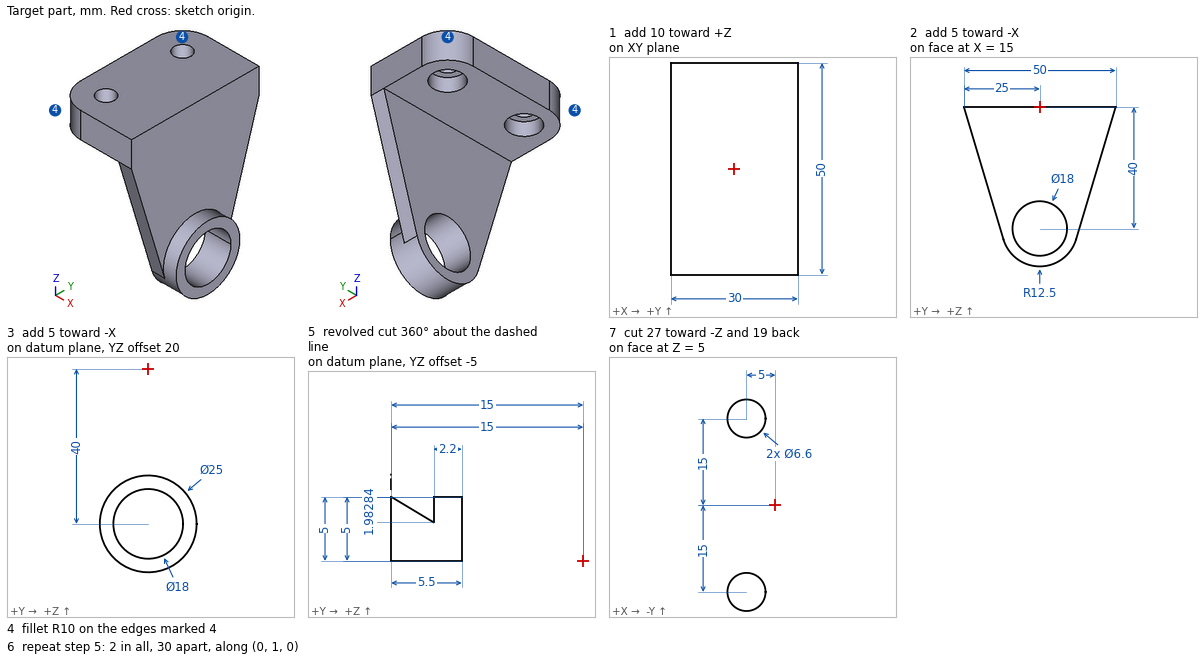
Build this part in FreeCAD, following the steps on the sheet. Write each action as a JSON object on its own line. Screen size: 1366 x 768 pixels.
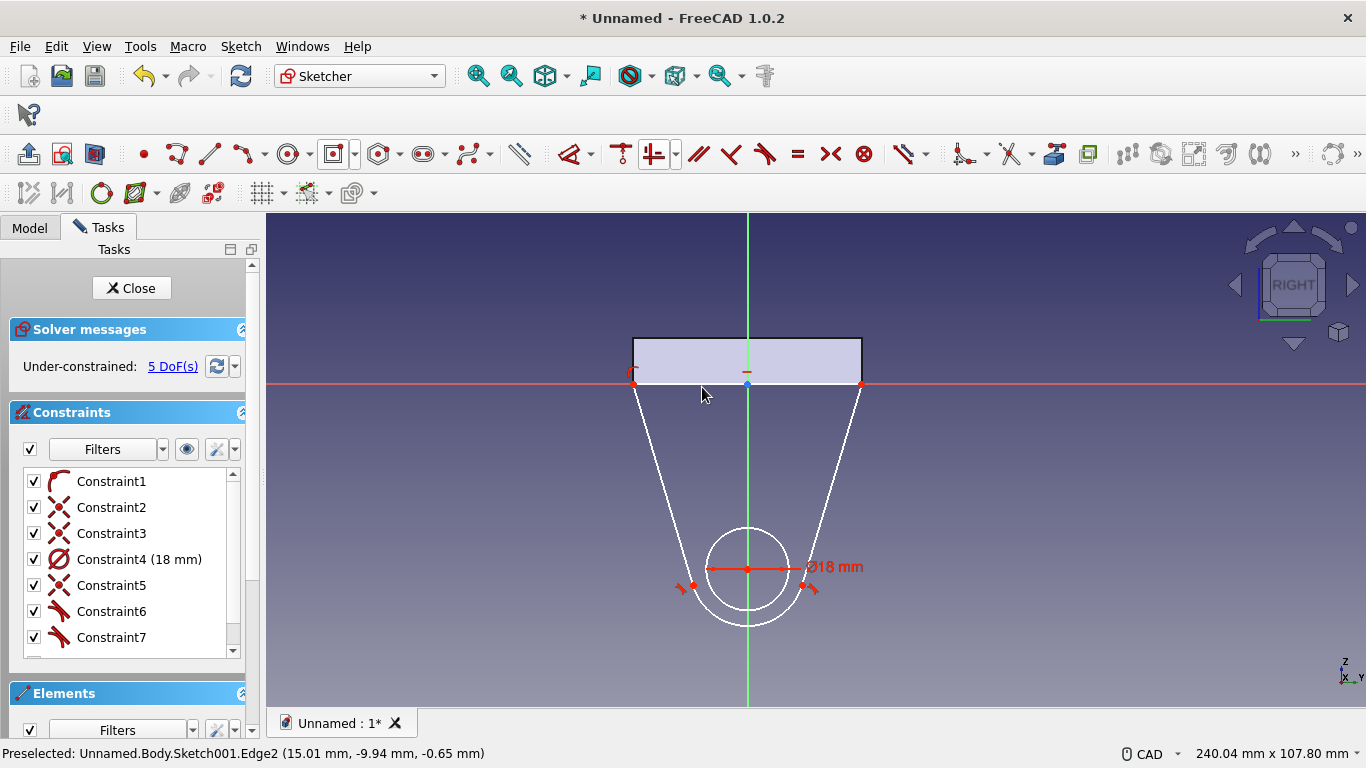
{"action": "left_click", "coordinate": [748, 569]}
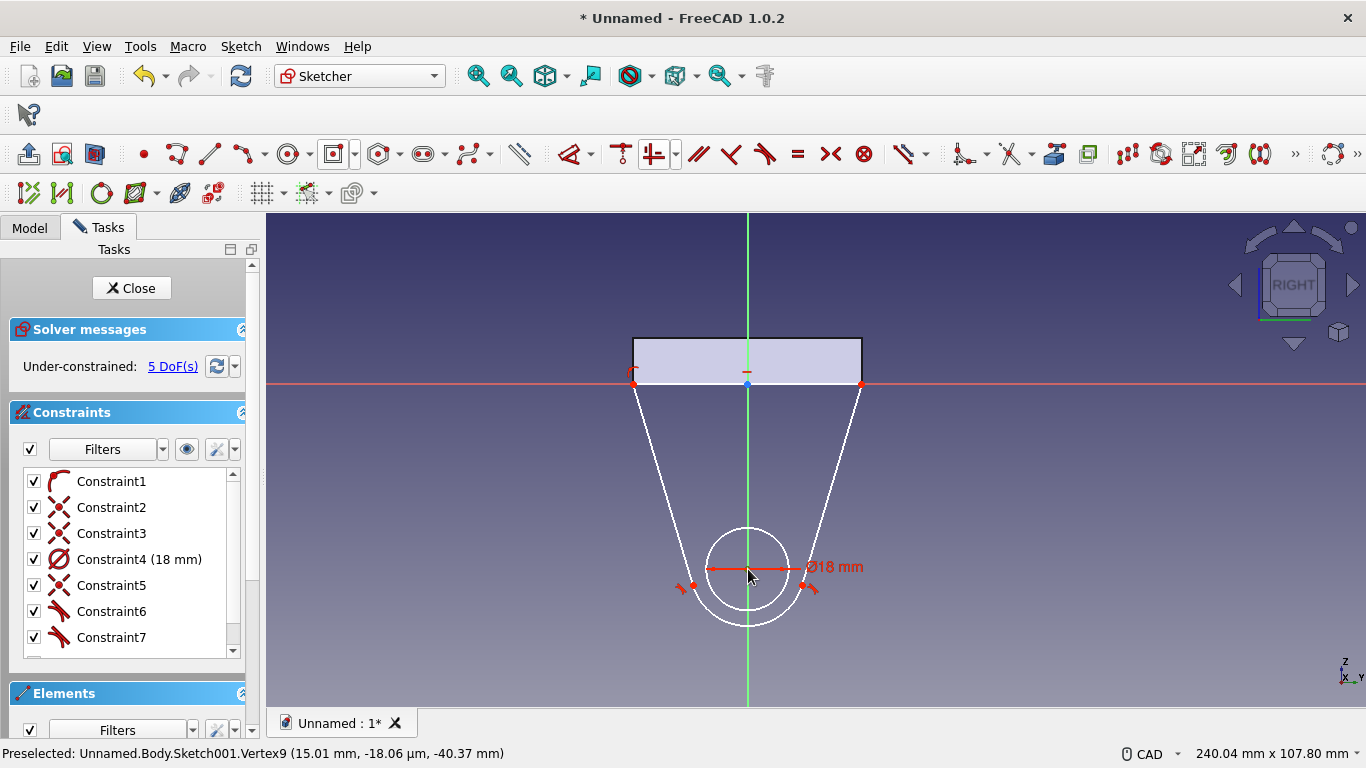
{"action": "left_click", "coordinate": [748, 491]}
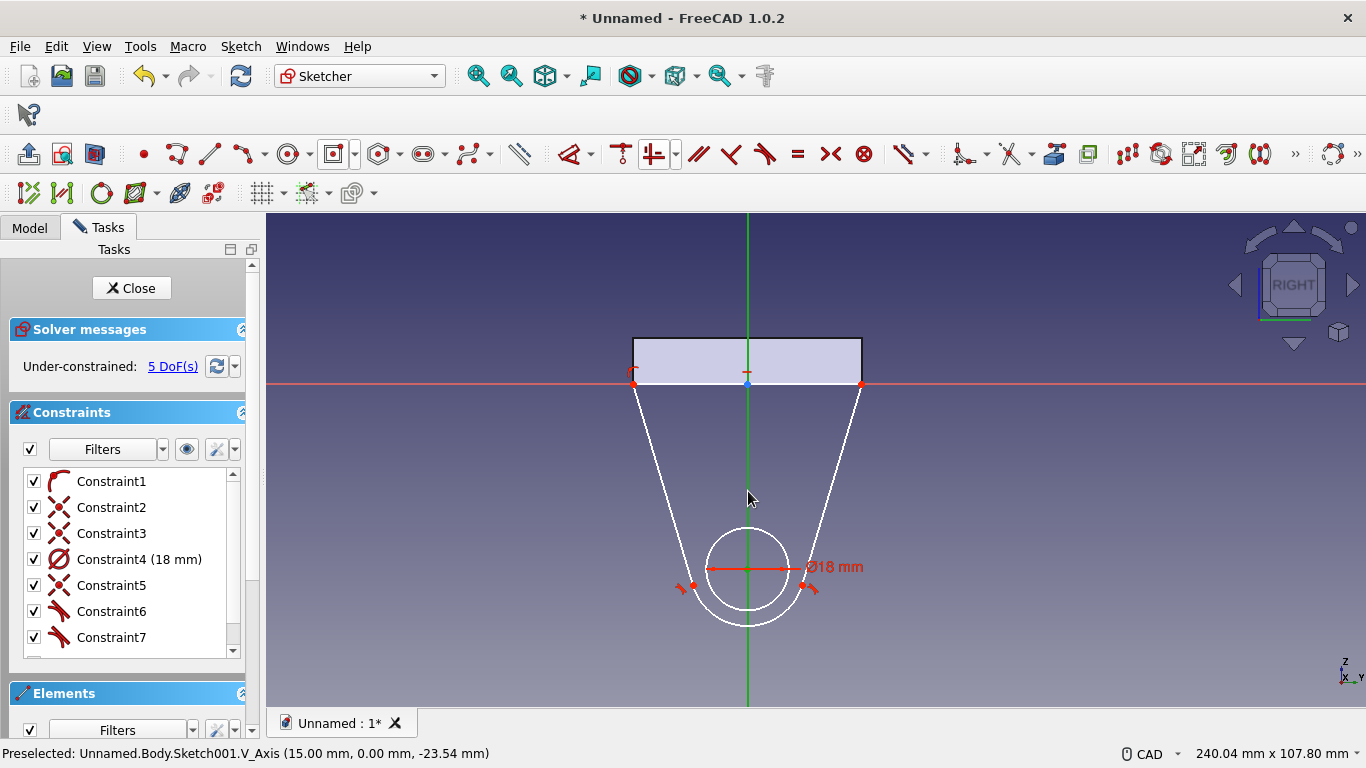
{"action": "left_click", "coordinate": [621, 154]}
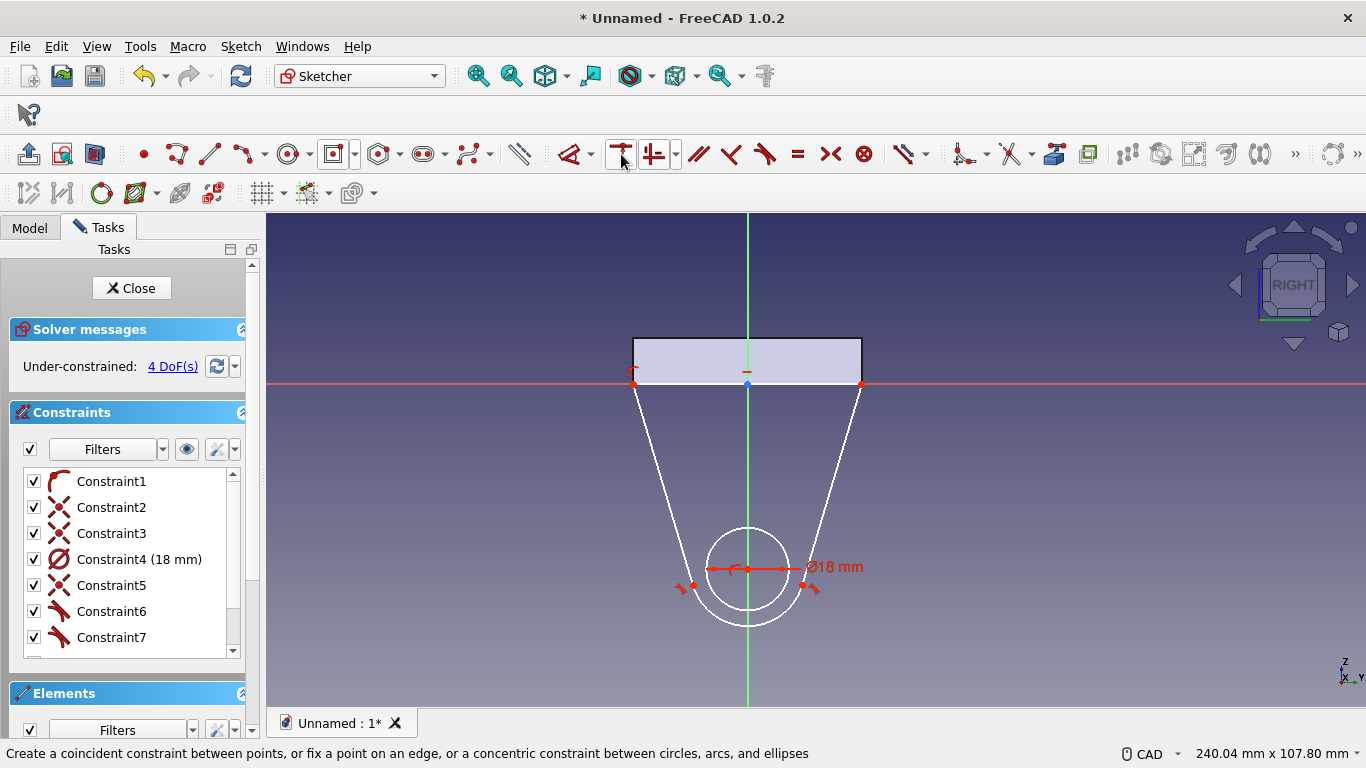
{"action": "left_click", "coordinate": [568, 154]}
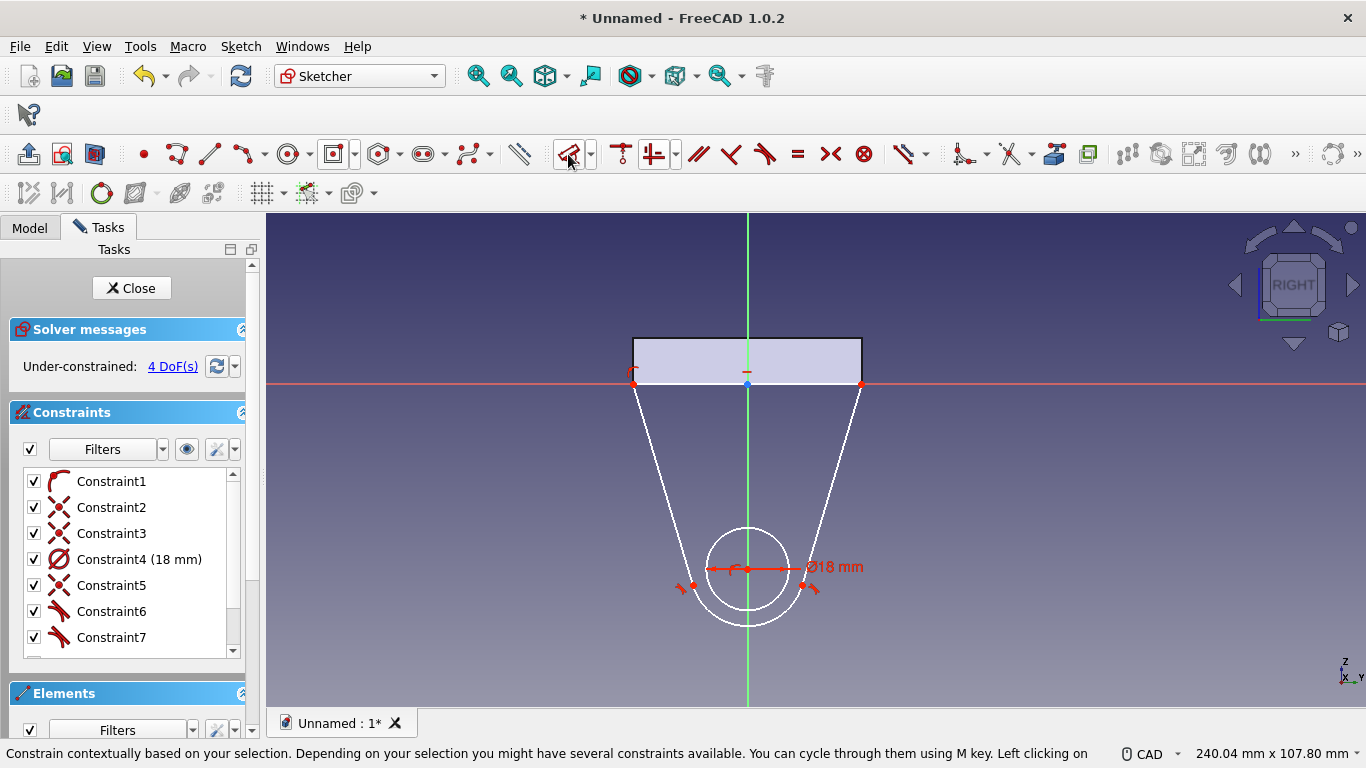
{"action": "left_click", "coordinate": [720, 619]}
{"action": "left_click", "coordinate": [705, 647]}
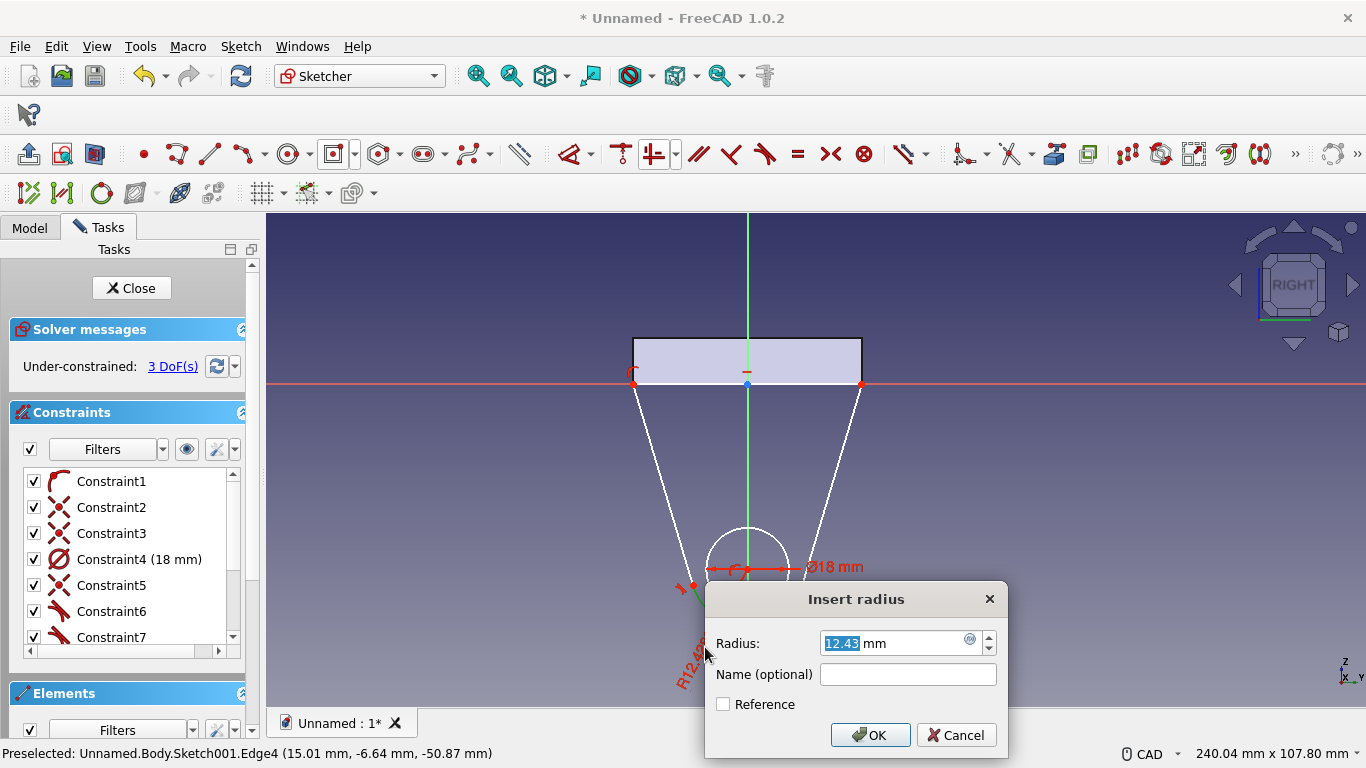
{"action": "type", "text": "12.5"}
{"action": "key", "text": "Return"}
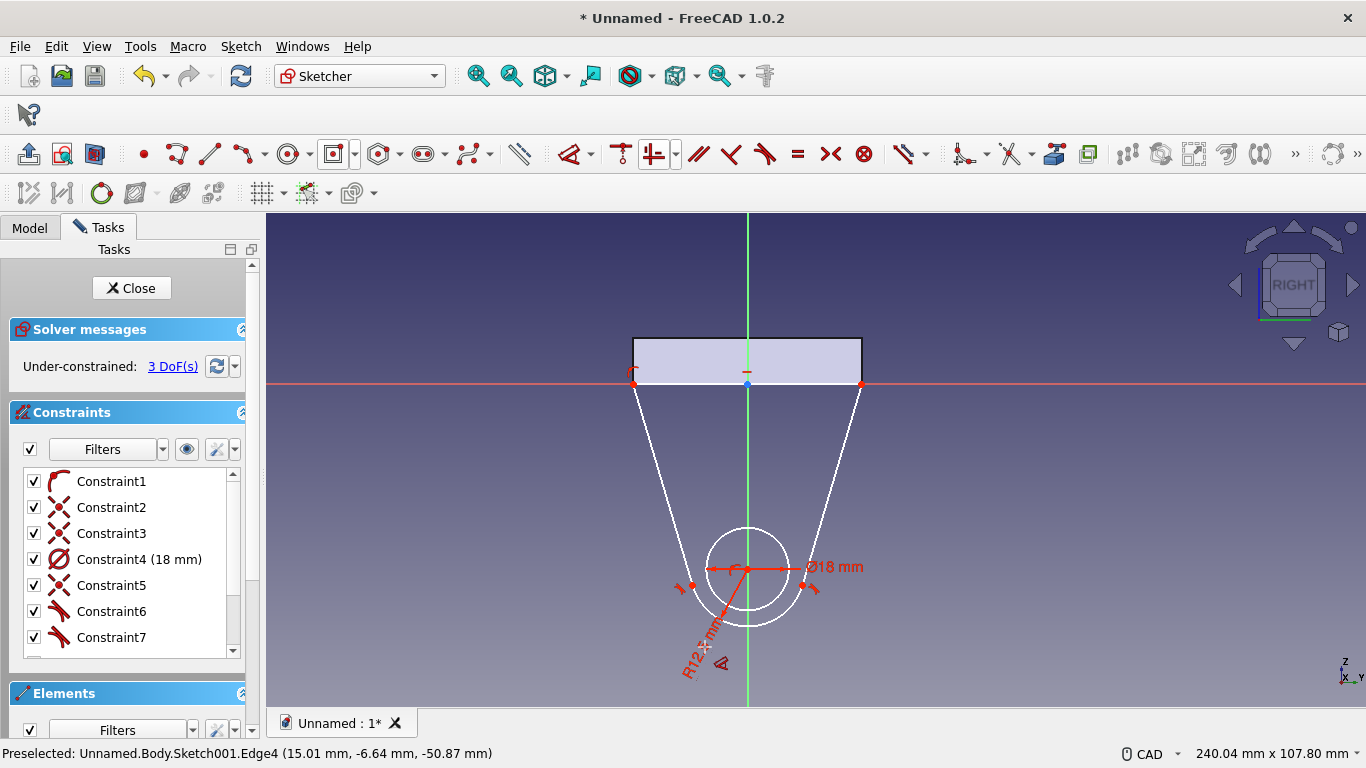
{"action": "left_click", "coordinate": [702, 384]}
{"action": "left_click", "coordinate": [695, 350]}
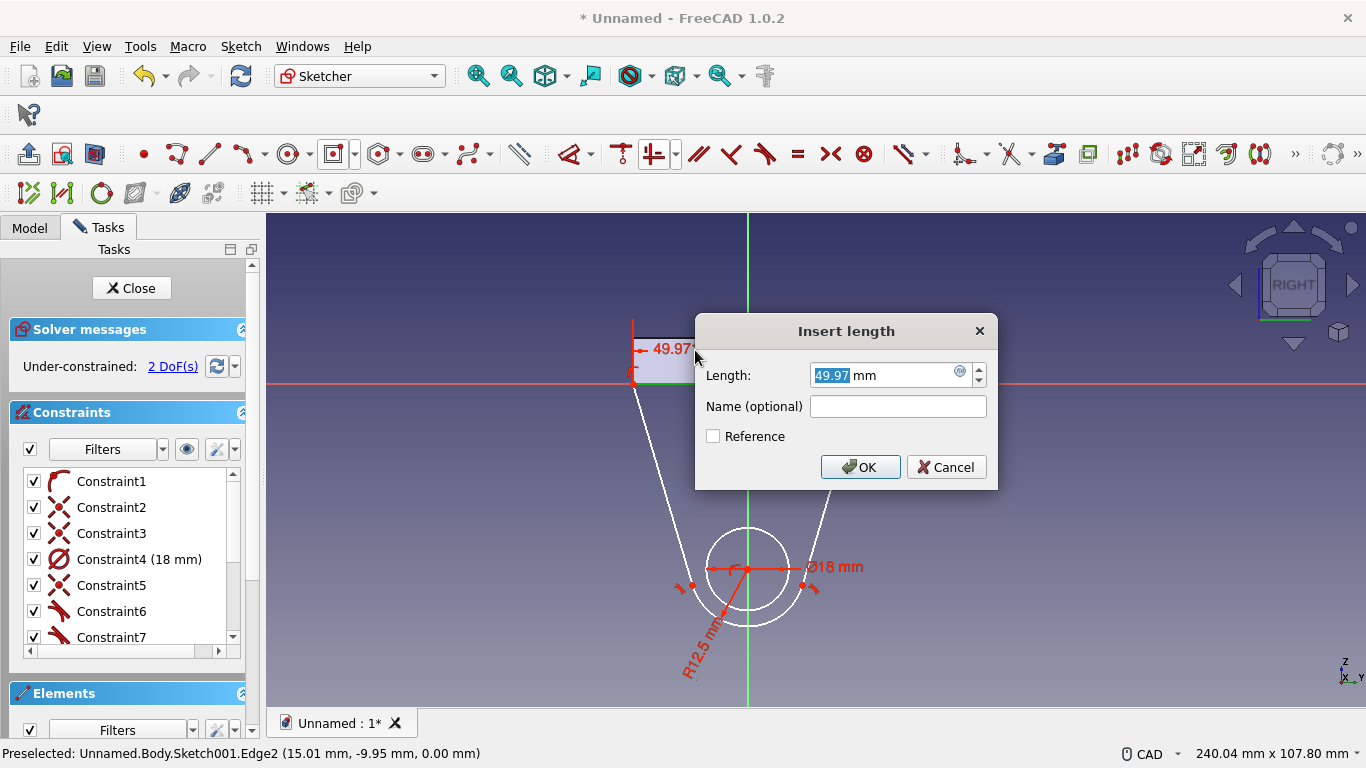
{"action": "type", "text": "50"}
{"action": "key", "text": "Return"}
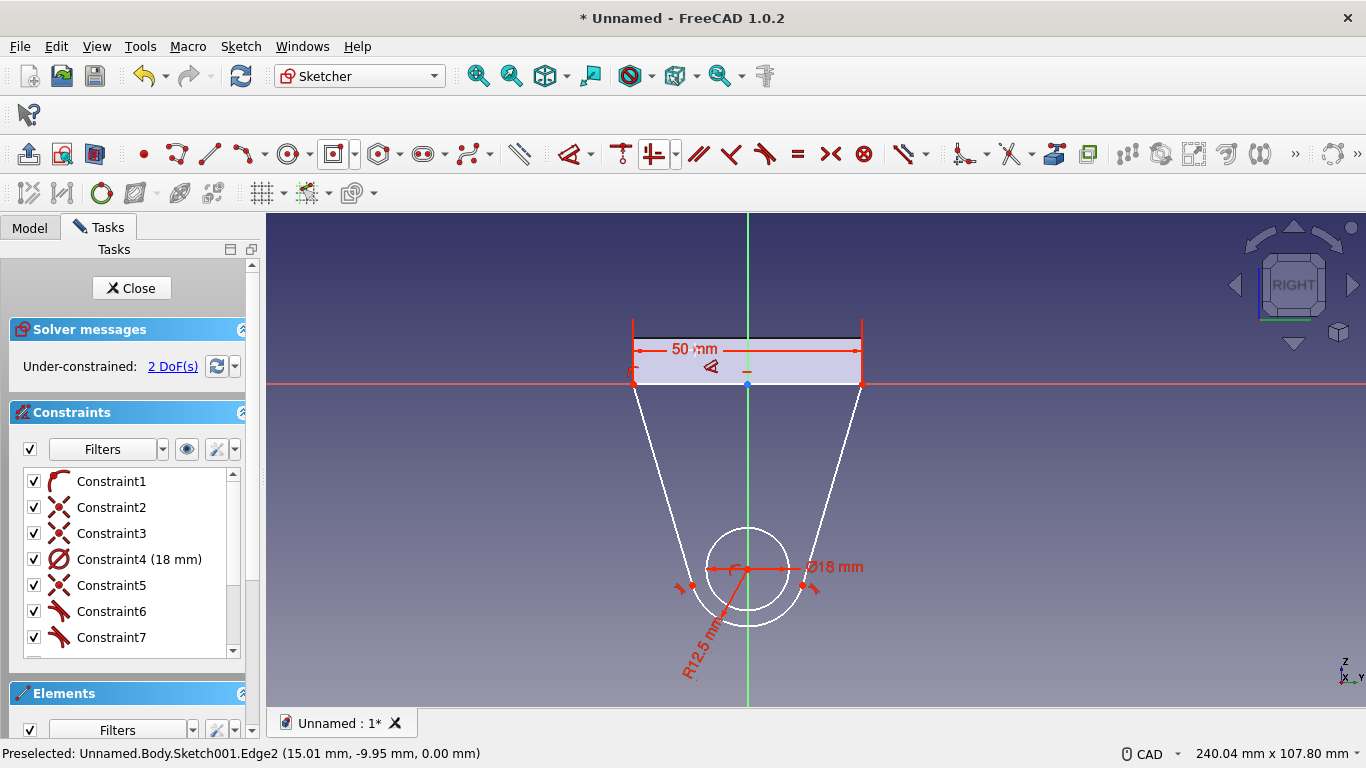
{"action": "left_click", "coordinate": [748, 569]}
{"action": "left_click", "coordinate": [782, 477]}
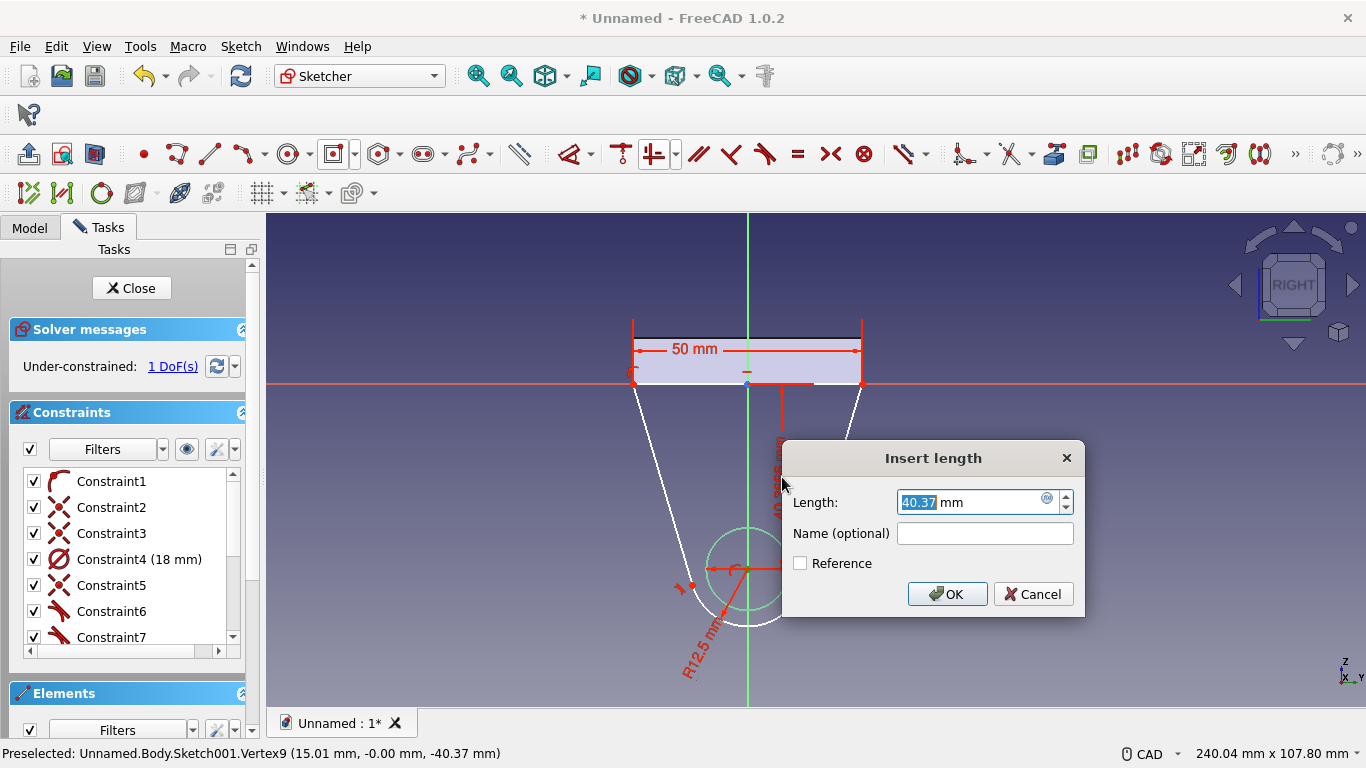
{"action": "type", "text": "40"}
{"action": "key", "text": "Return"}